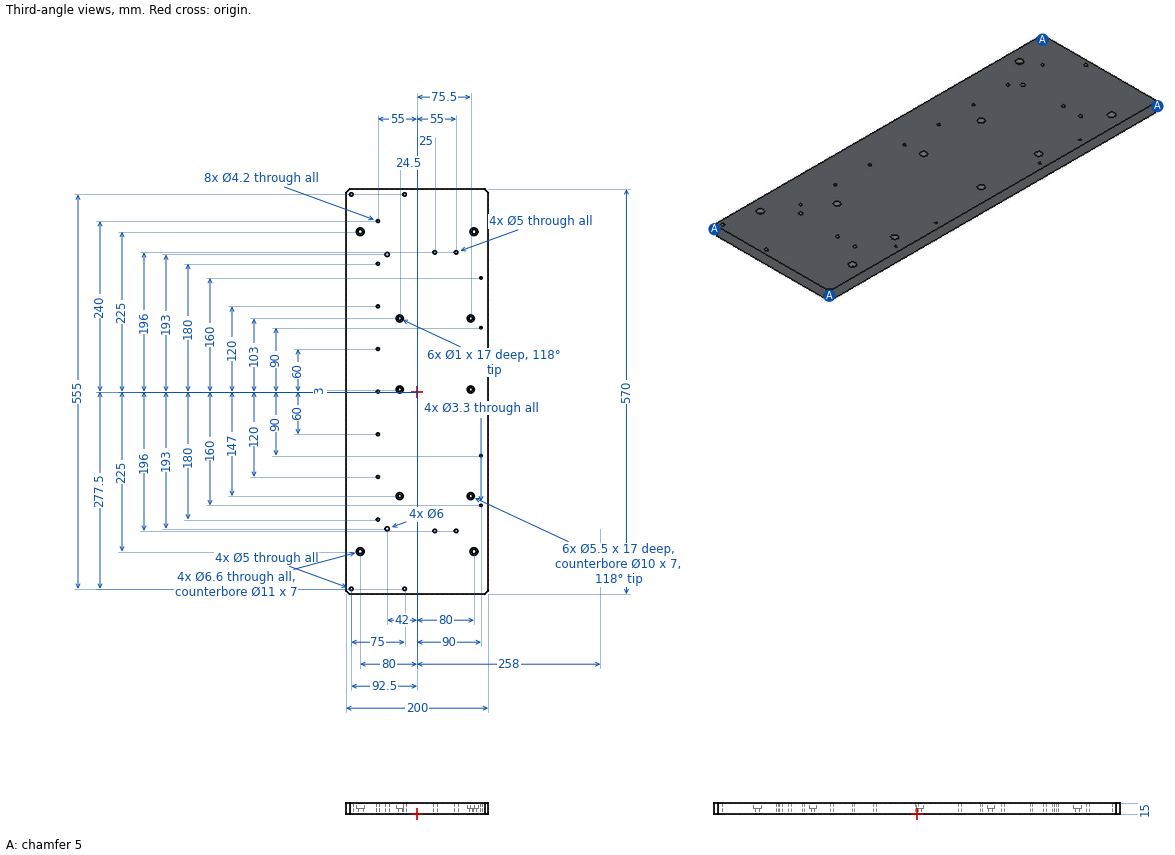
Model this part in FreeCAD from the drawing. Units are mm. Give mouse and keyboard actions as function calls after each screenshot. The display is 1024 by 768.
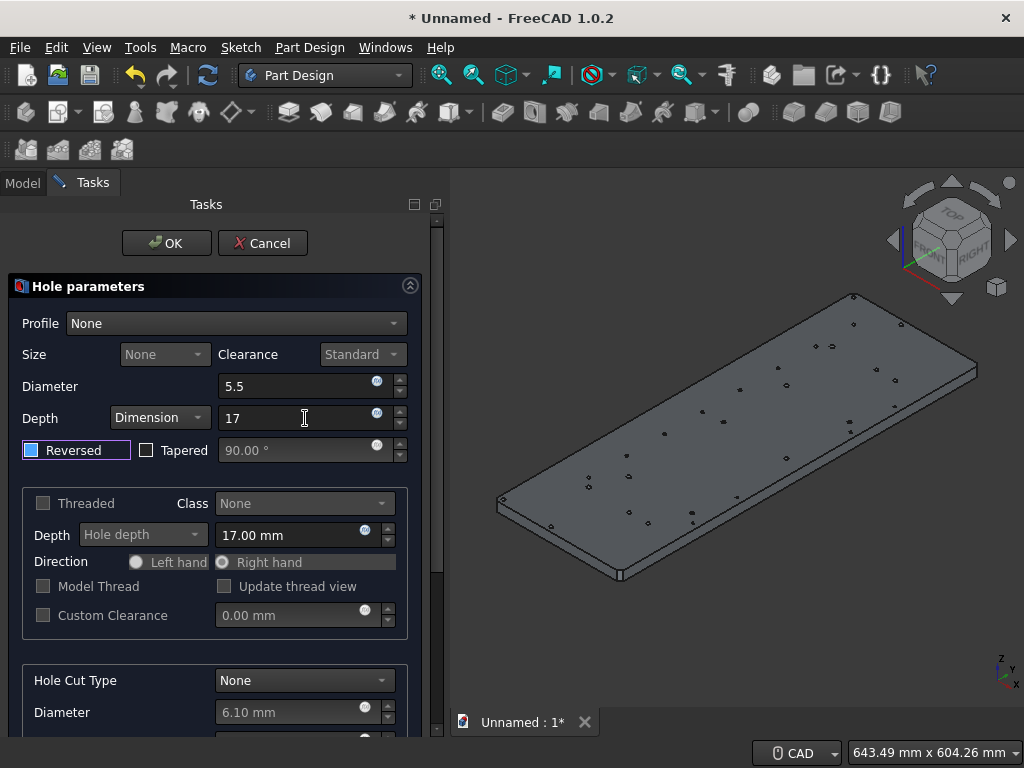
click(306, 680)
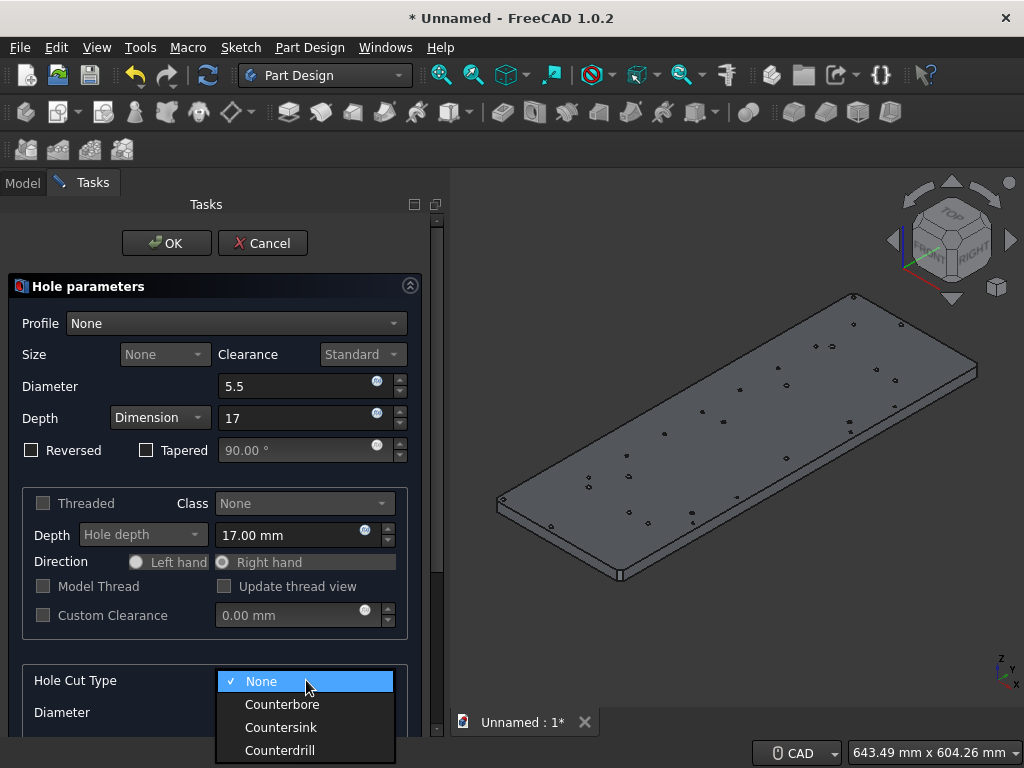
click(304, 704)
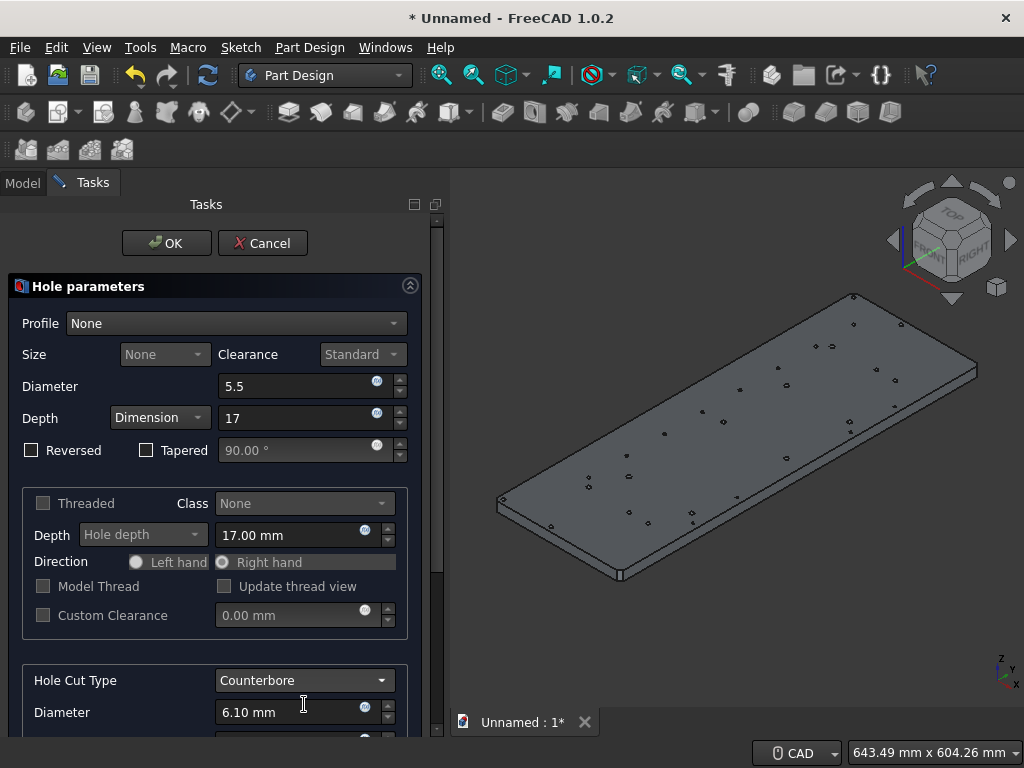
triple_click(298, 712)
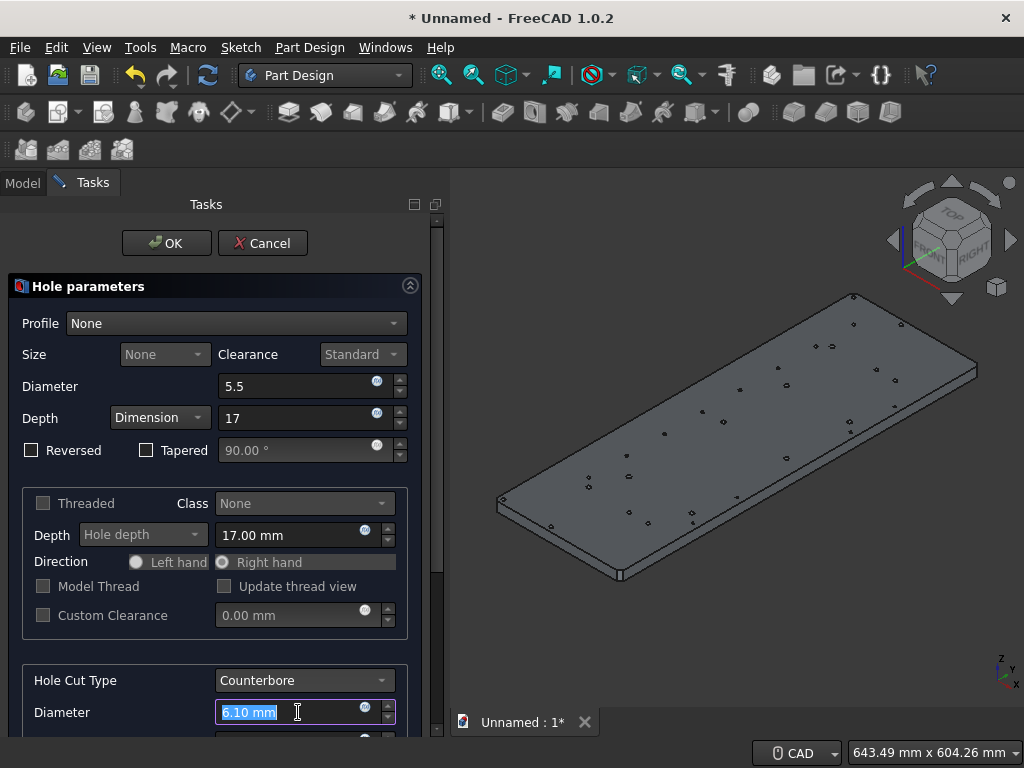
text(10)
key(Tab)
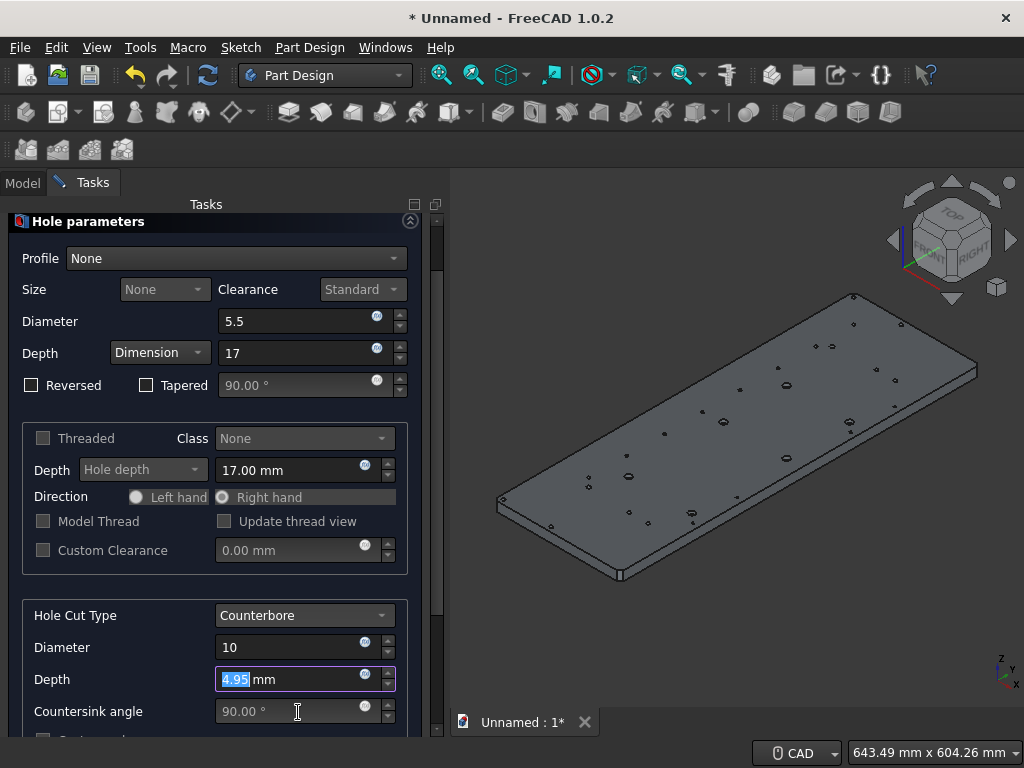
text(7)
key(Tab)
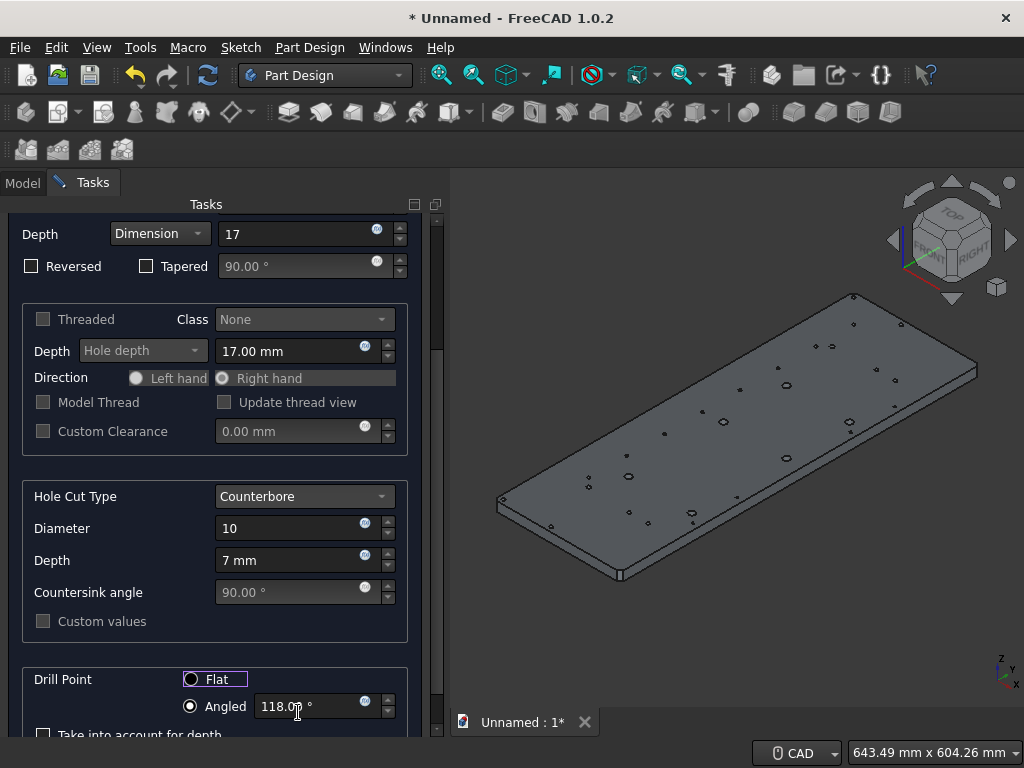
scroll(437, 475, up, 4)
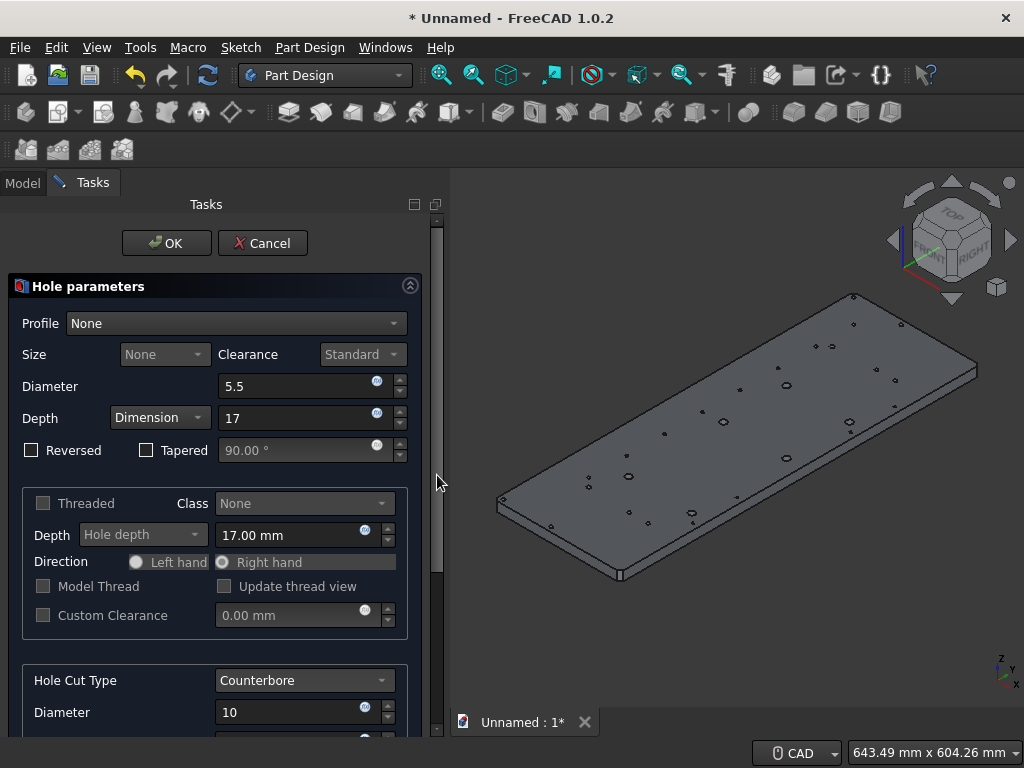
click(167, 243)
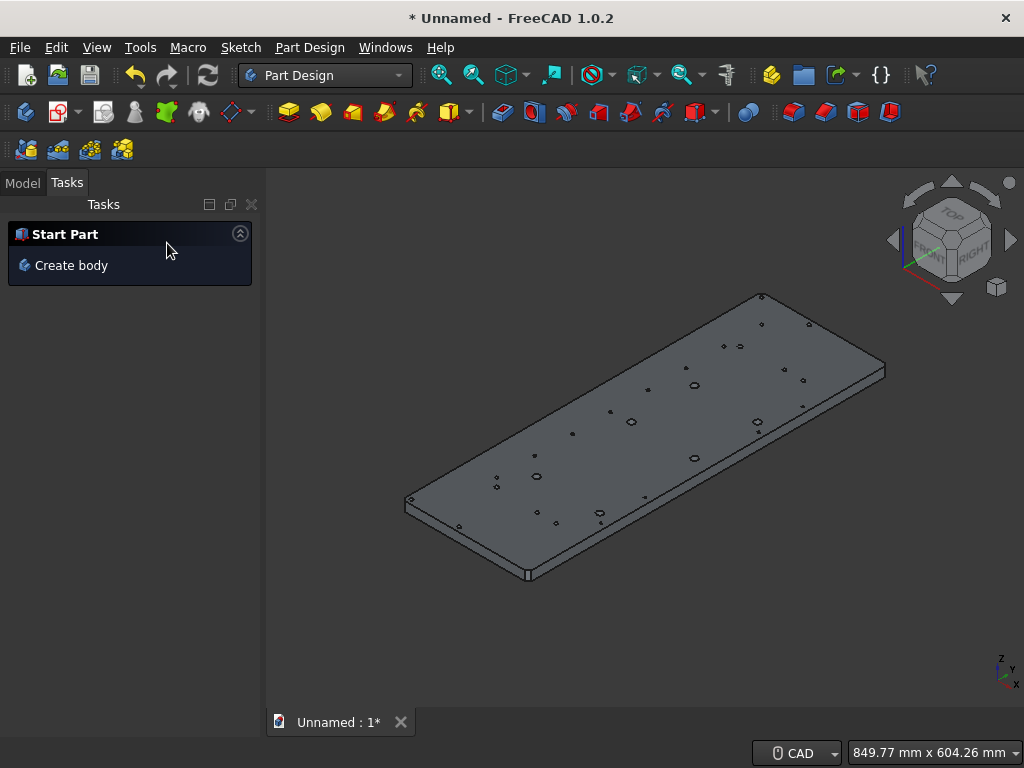
click(612, 471)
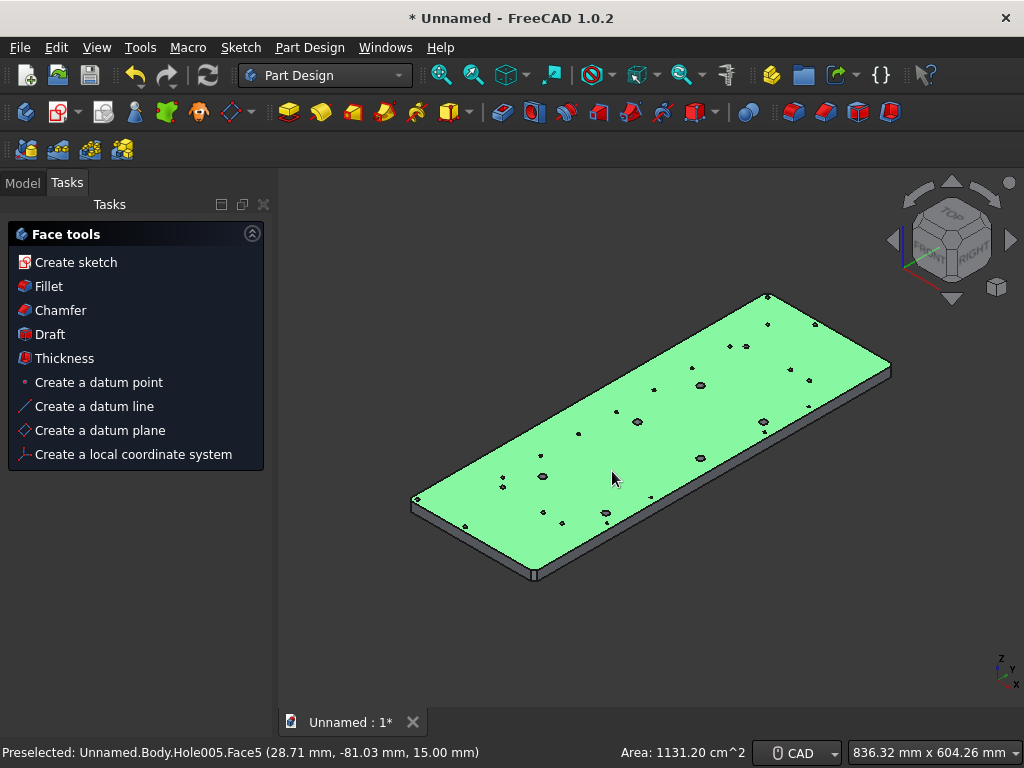
click(58, 112)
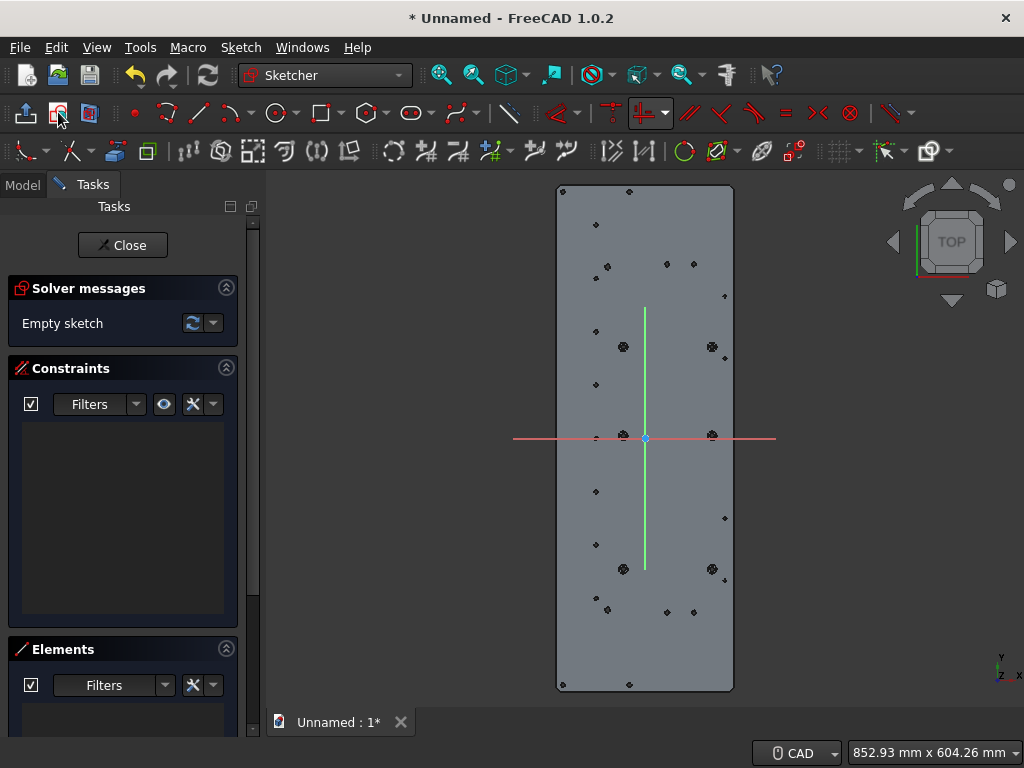
click(276, 114)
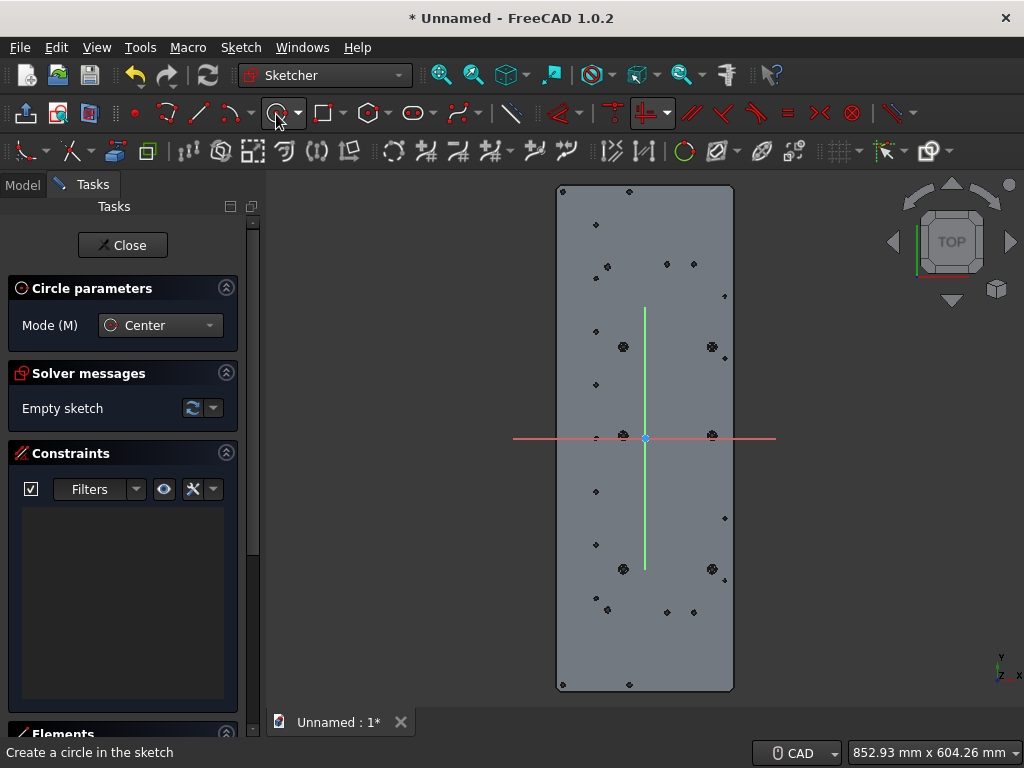
scroll(574, 638, up, 11)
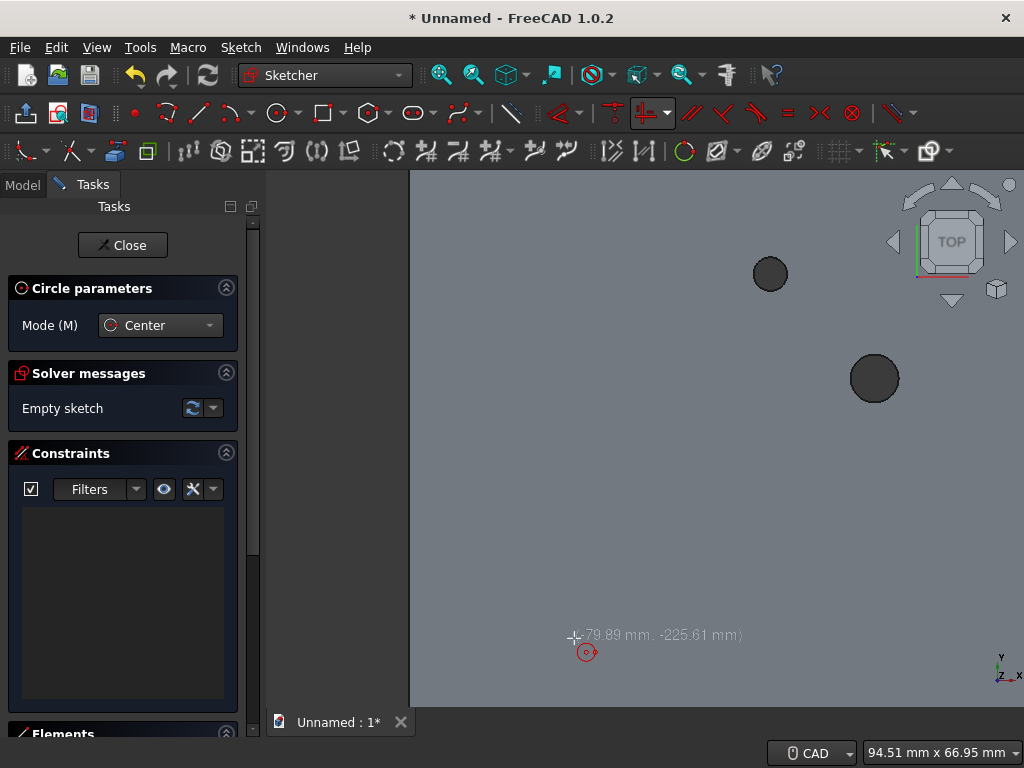
scroll(513, 599, down, 12)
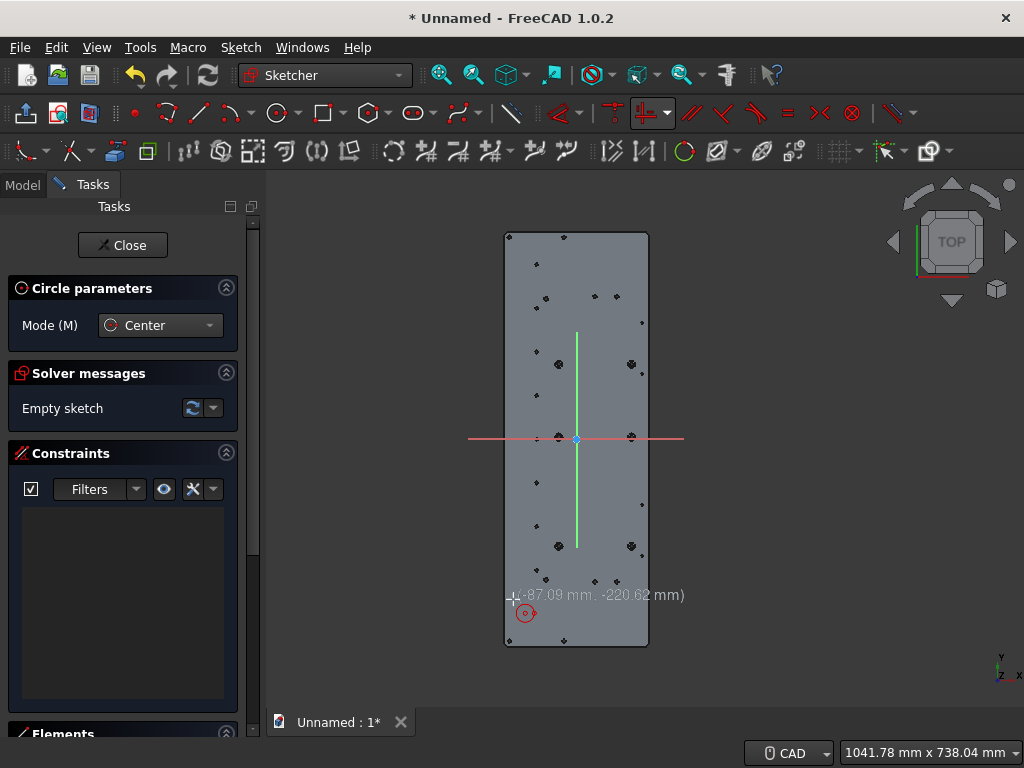
click(518, 603)
move(520, 601)